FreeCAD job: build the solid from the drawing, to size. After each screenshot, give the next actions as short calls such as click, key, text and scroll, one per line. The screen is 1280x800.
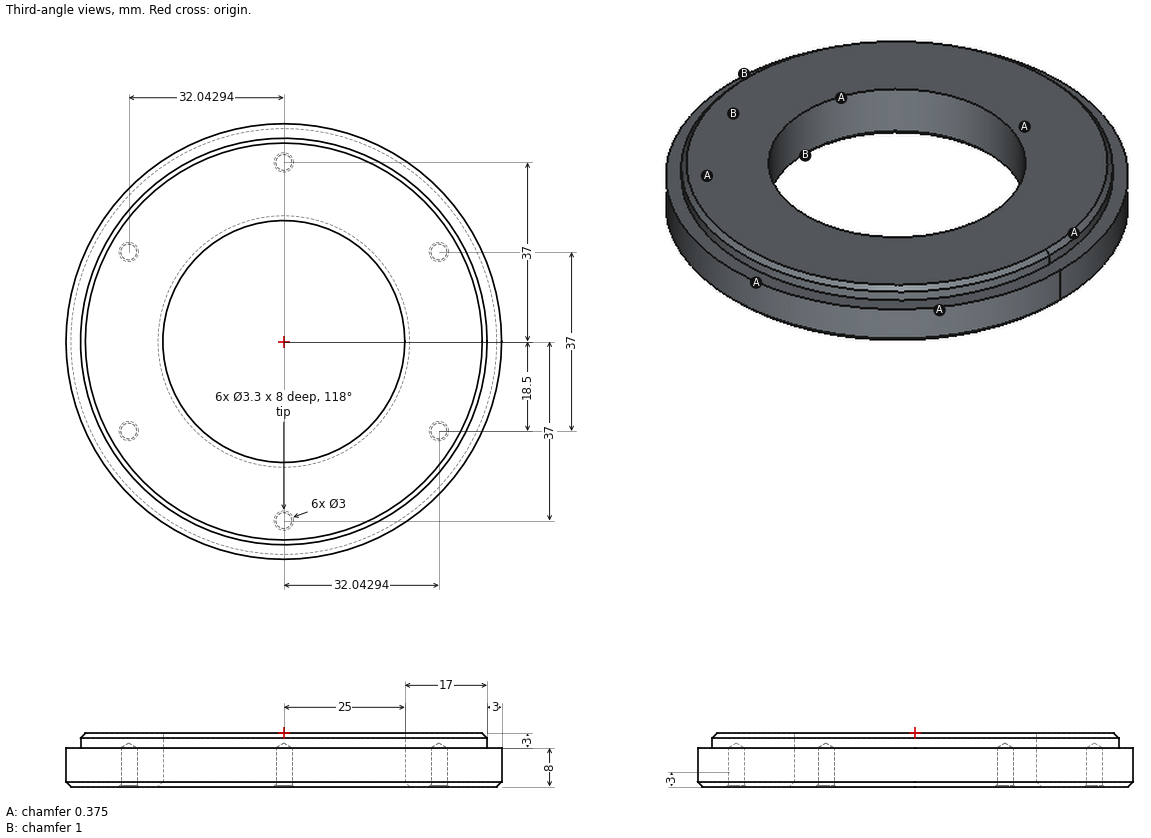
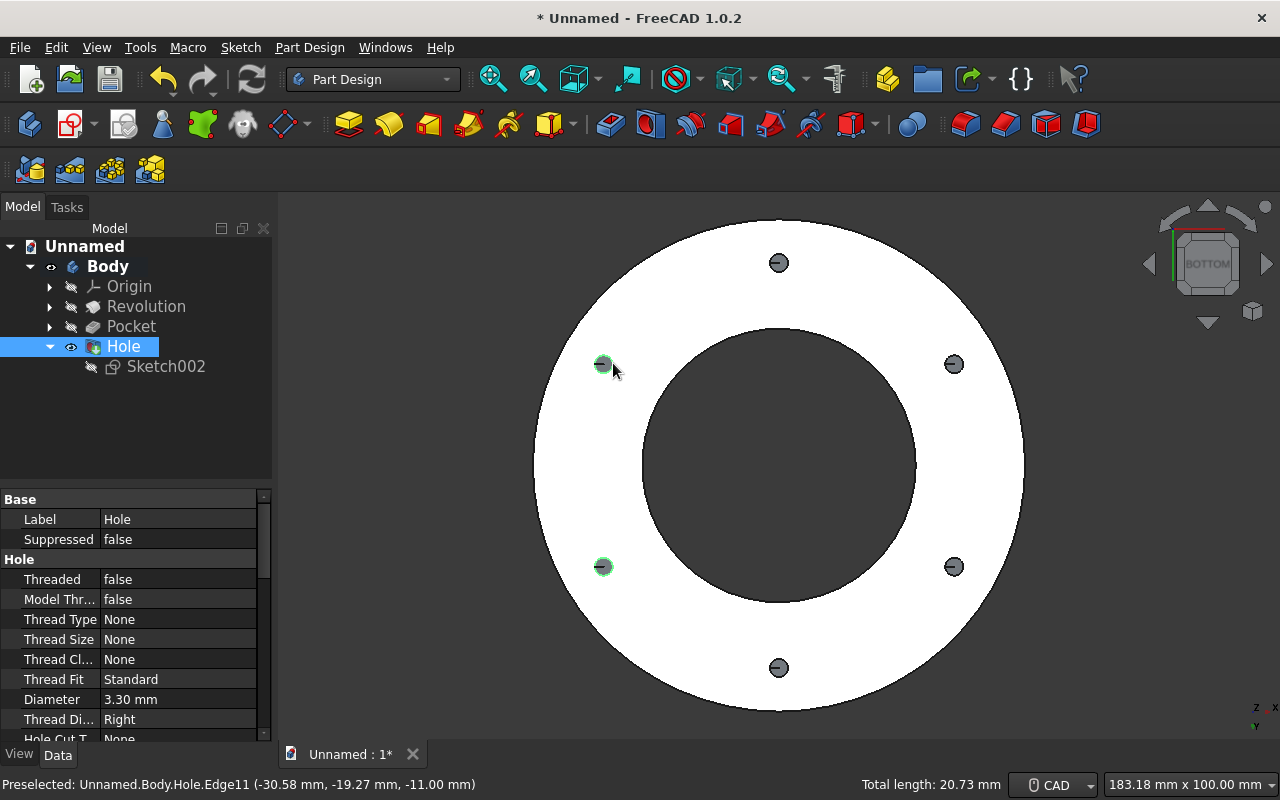
click(788, 667, ctrl)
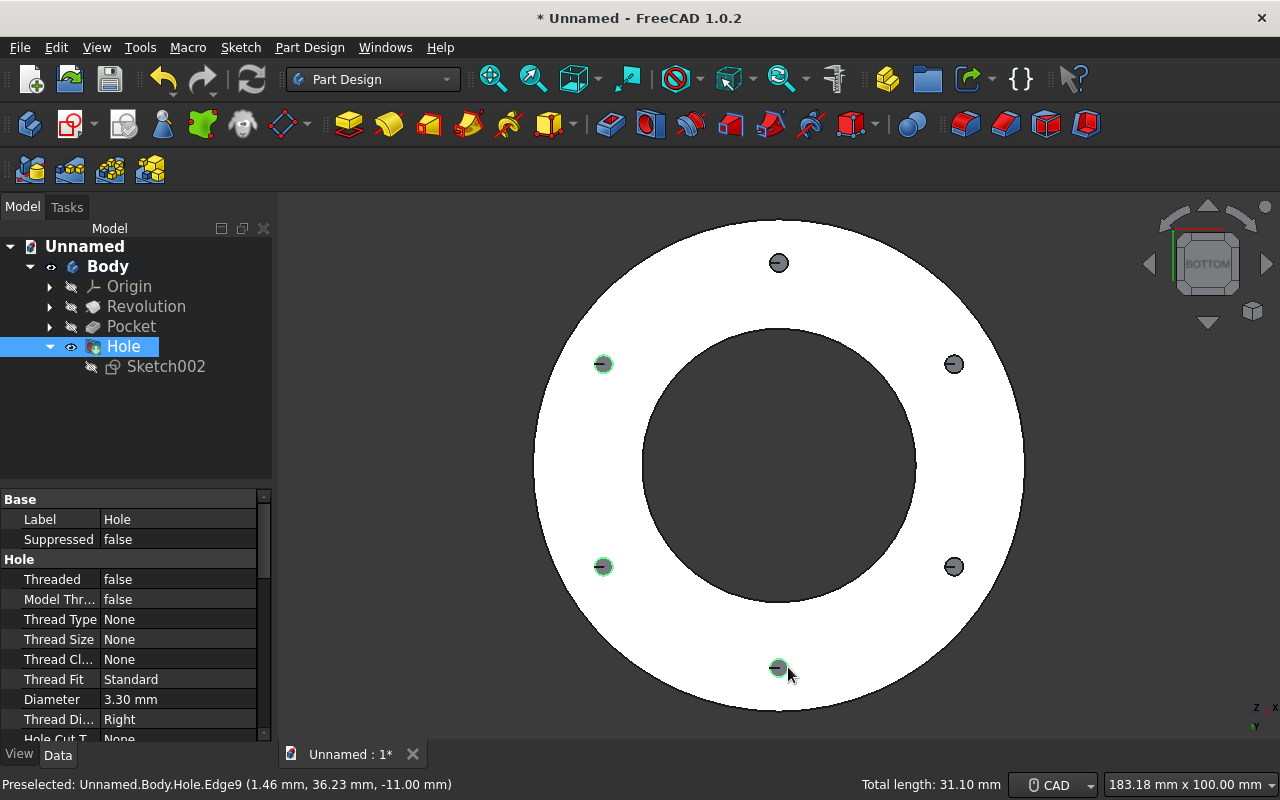
click(963, 566, ctrl)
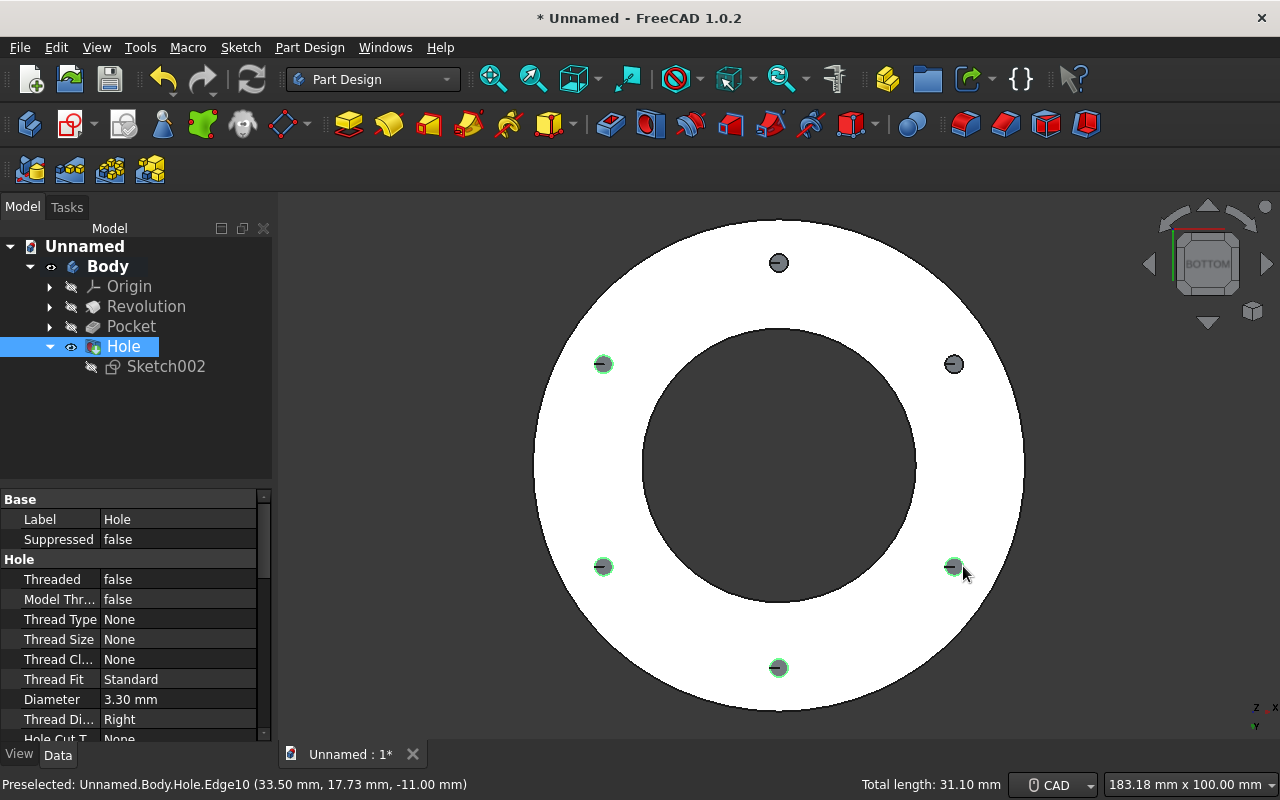
click(963, 363, ctrl)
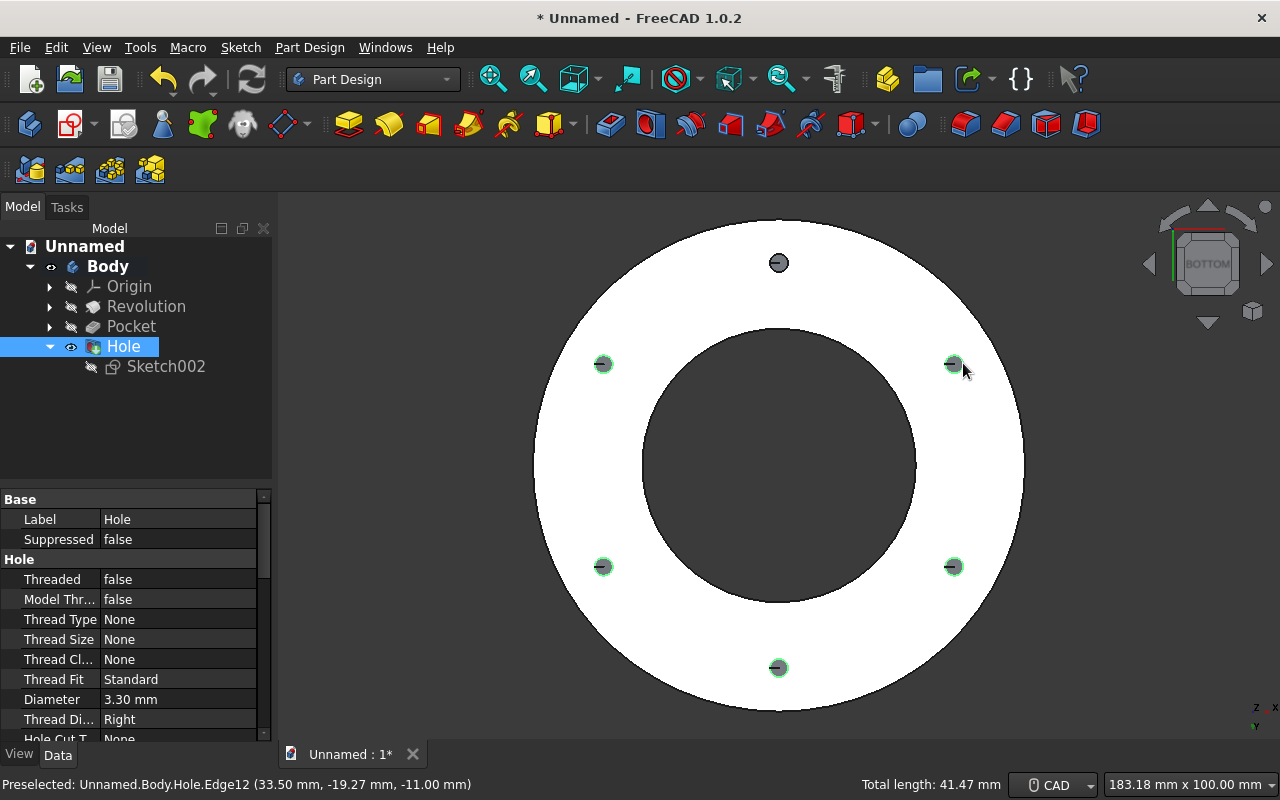
click(788, 262, ctrl)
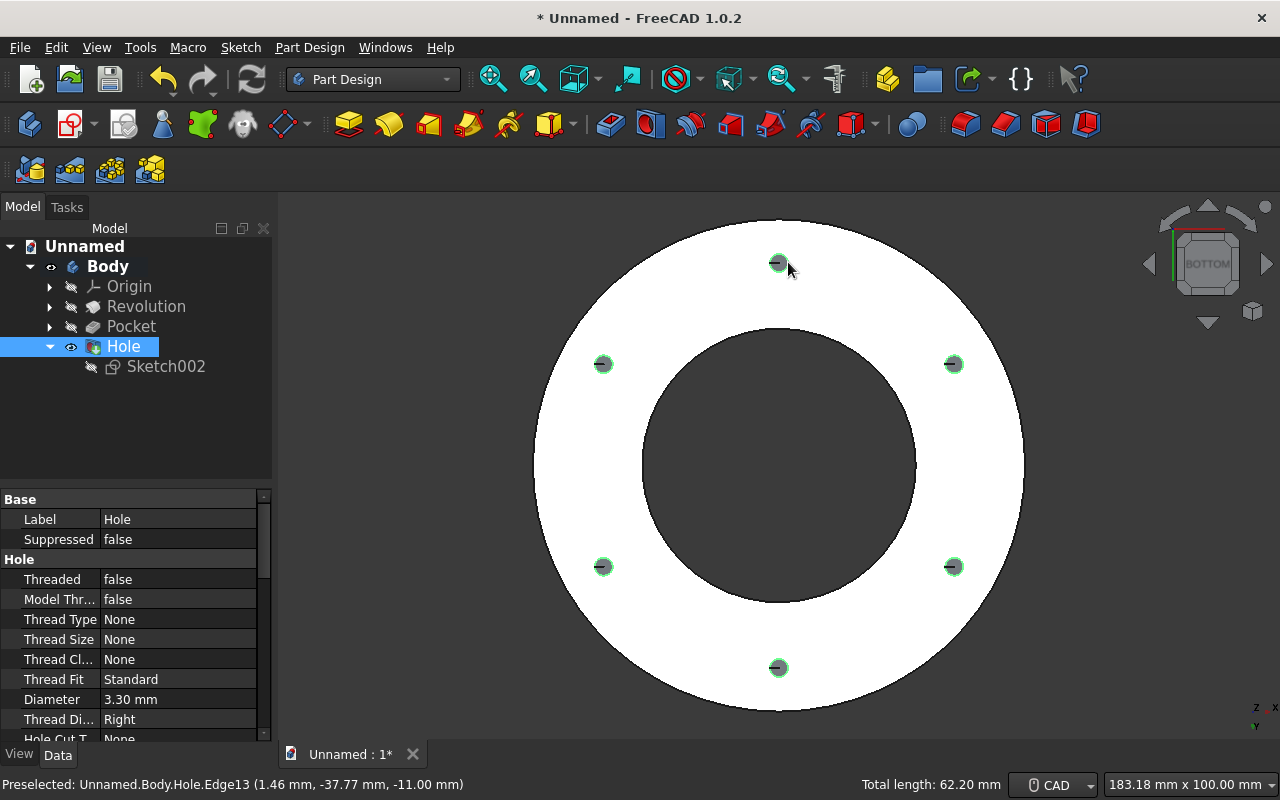
click(1006, 124)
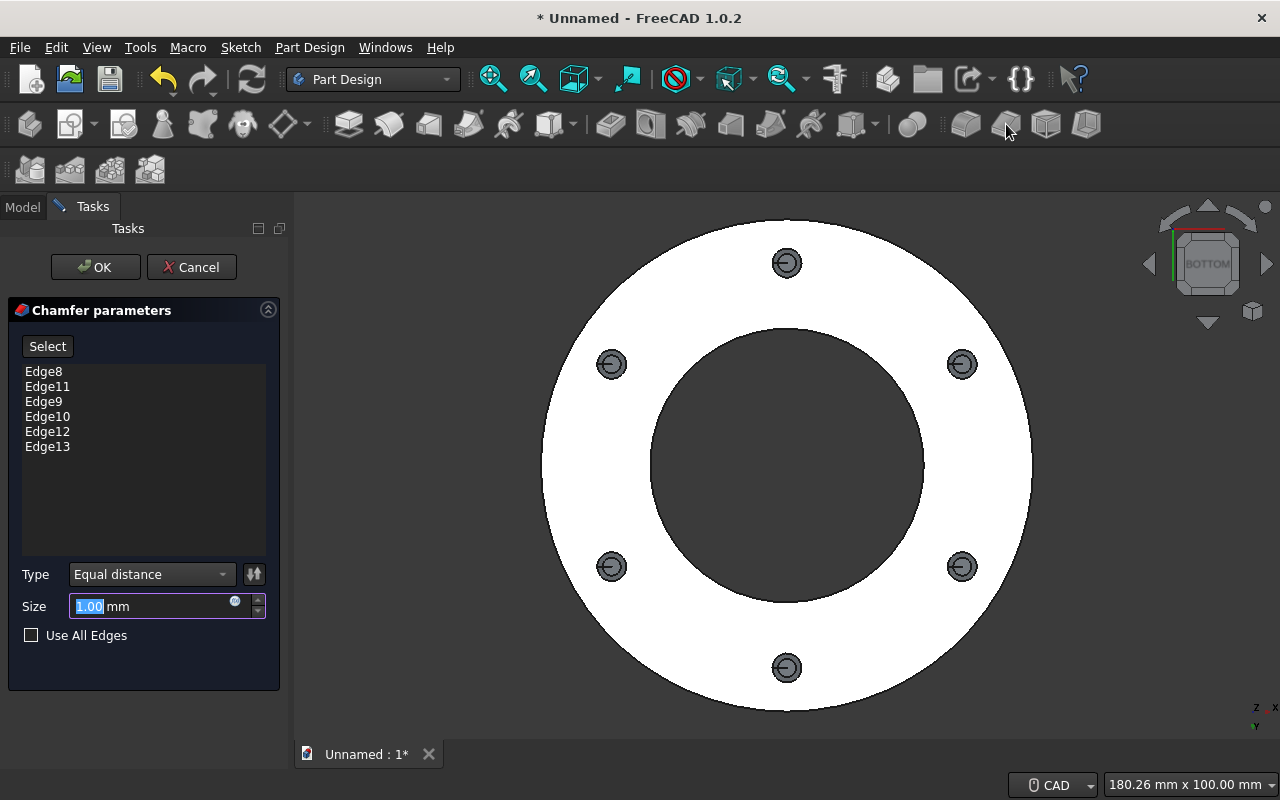
text(0.375)
key(Tab)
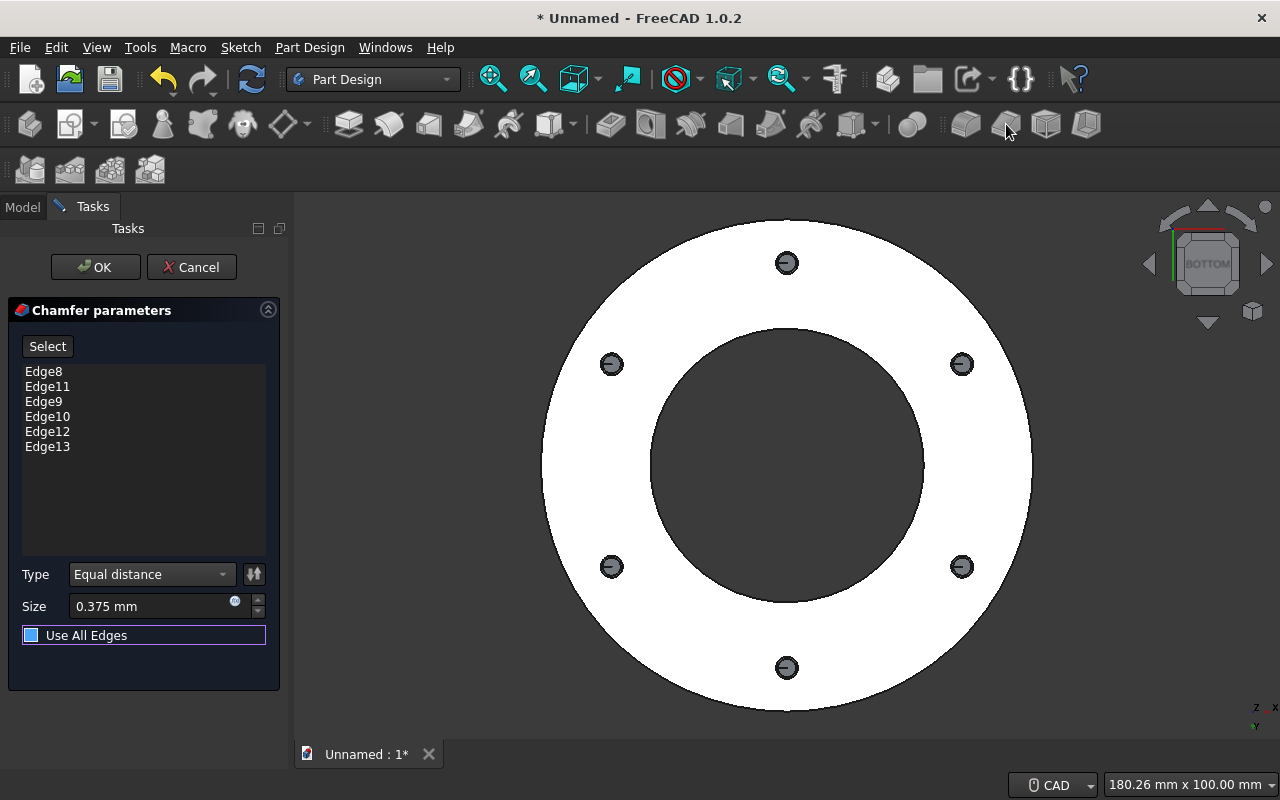
click(96, 267)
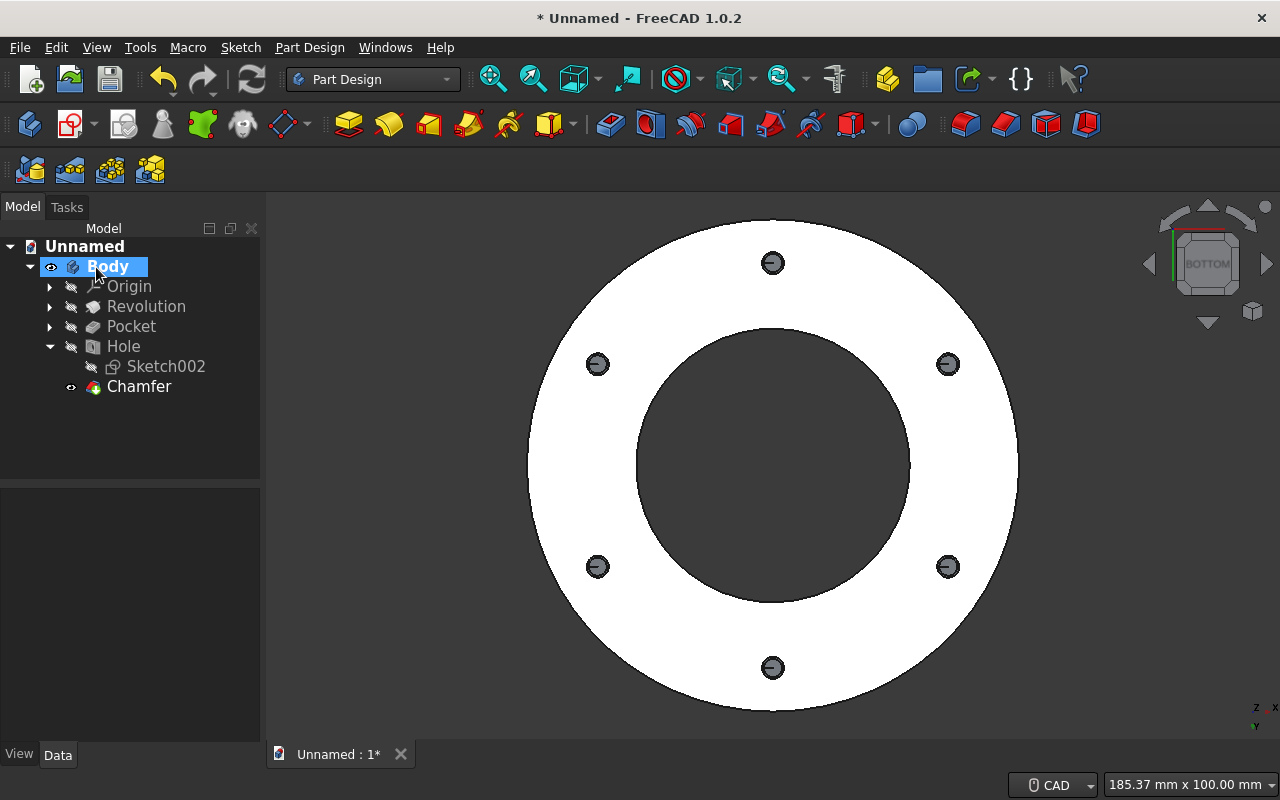
click(636, 465)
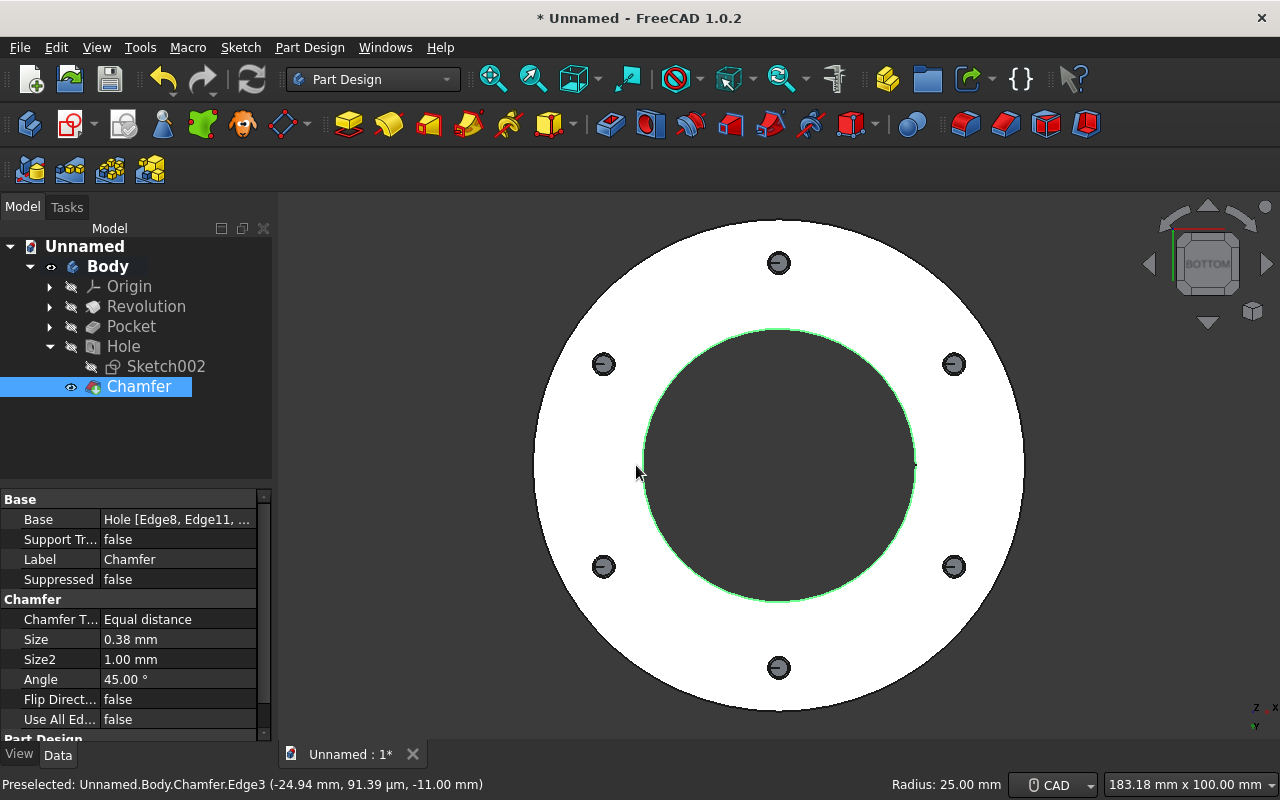
click(533, 465, ctrl)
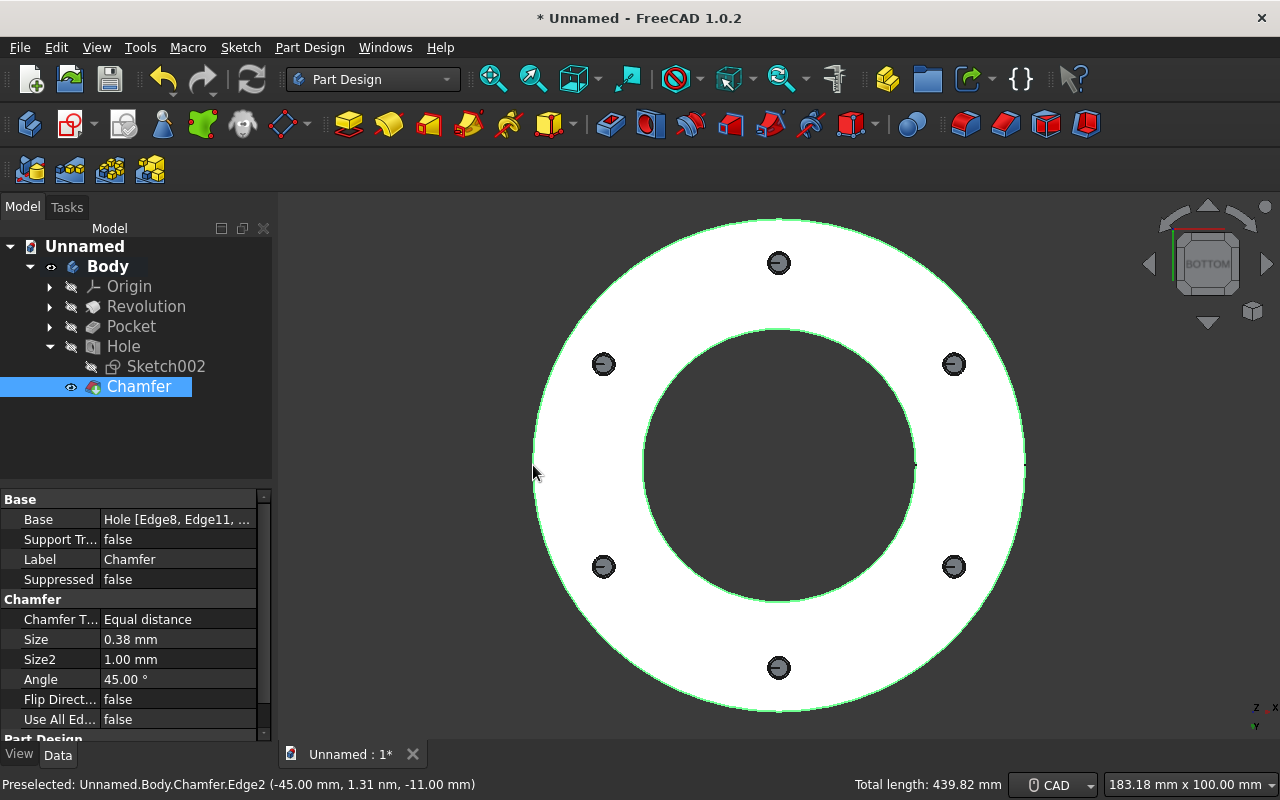
key(0)